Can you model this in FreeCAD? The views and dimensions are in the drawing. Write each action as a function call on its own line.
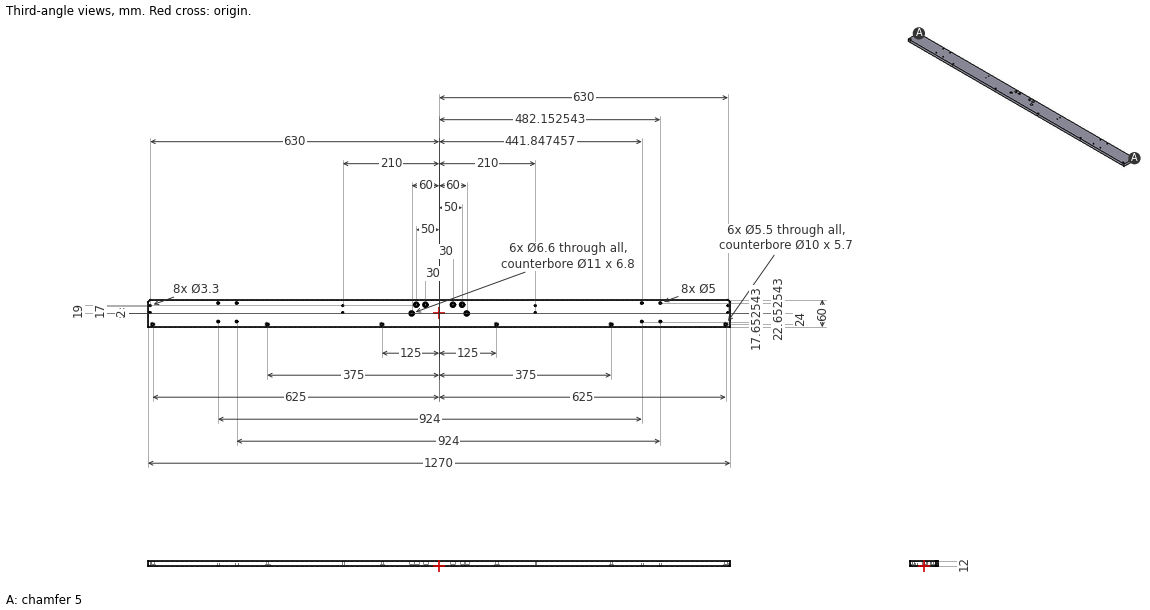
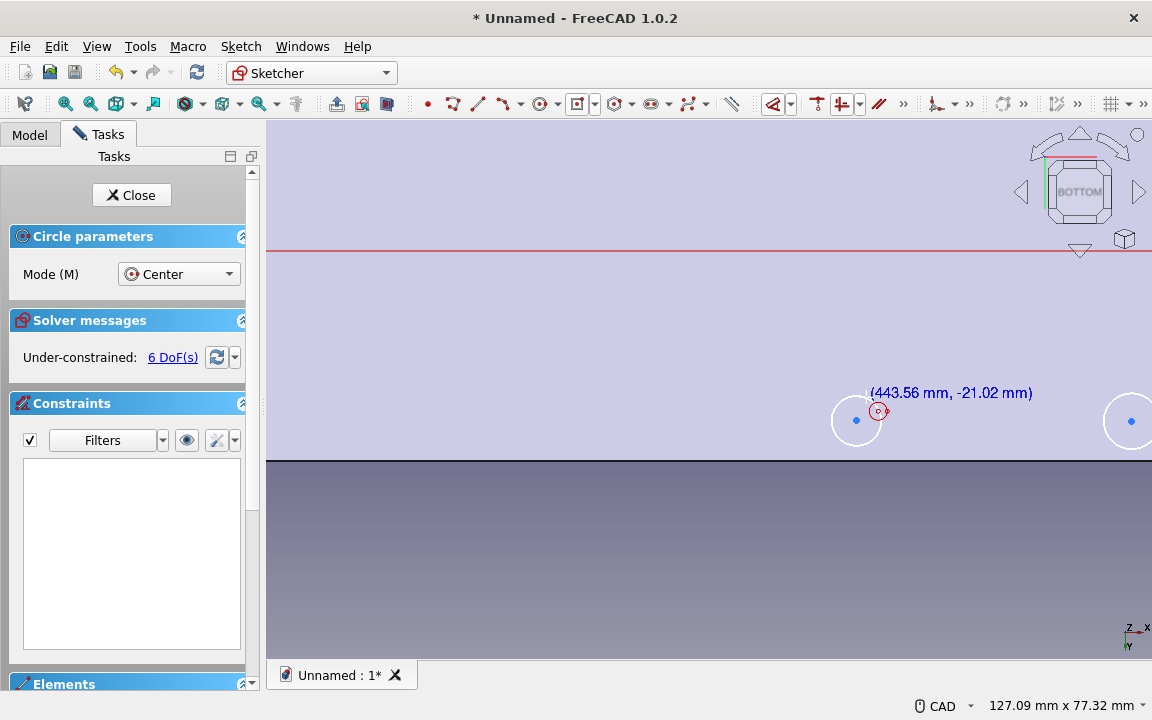
scroll(870, 399, down, 13)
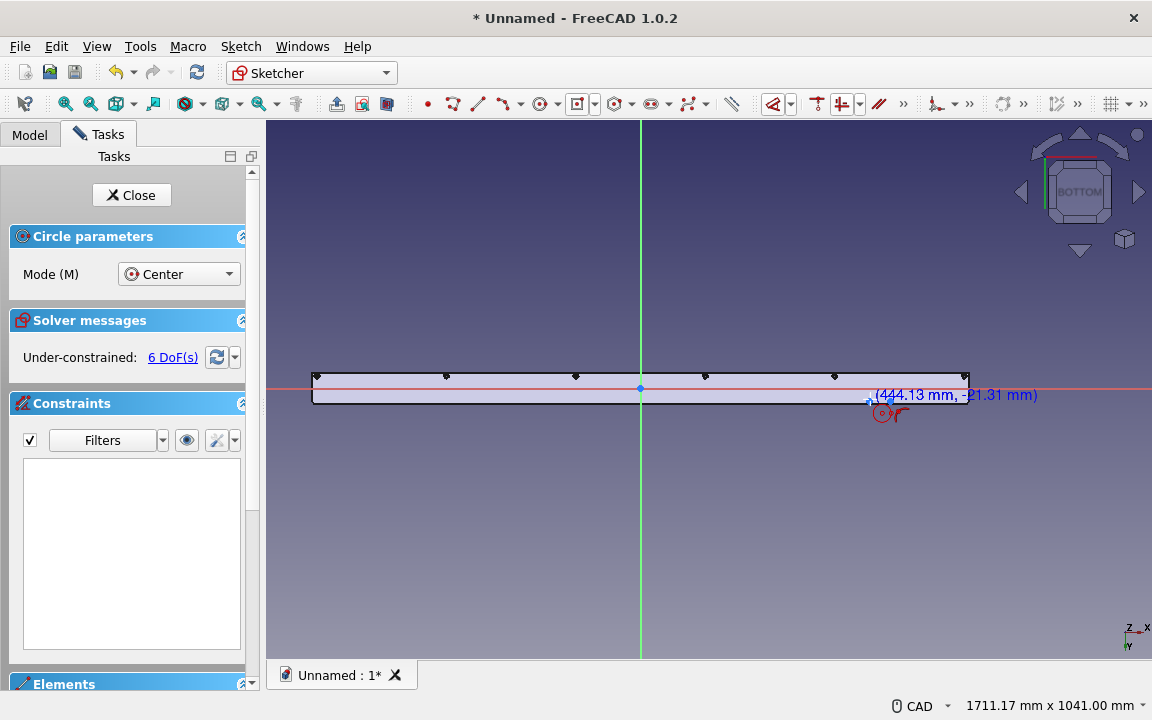
scroll(869, 379, up, 15)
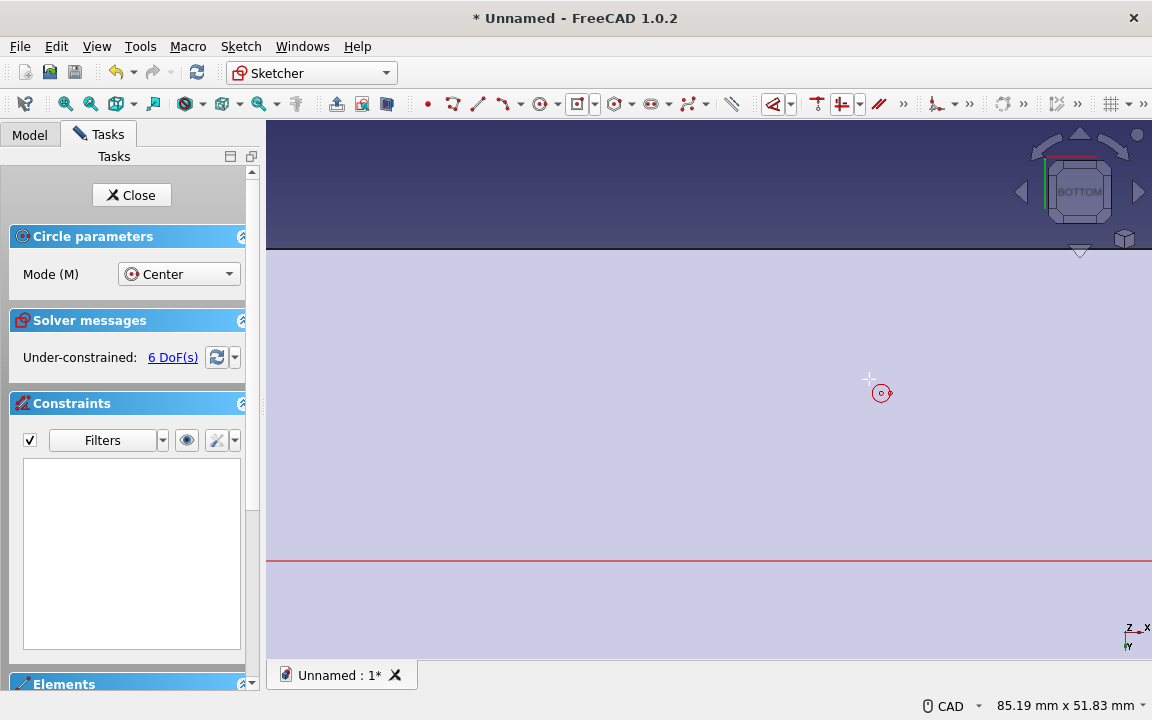
scroll(869, 379, down, 15)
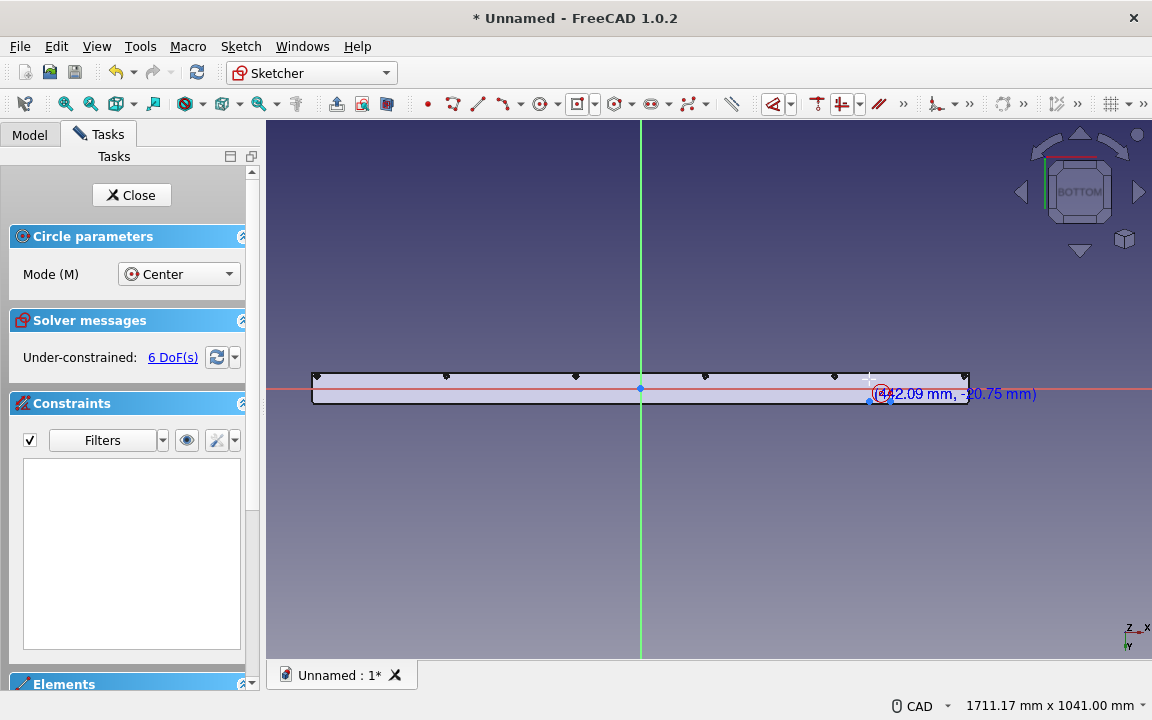
scroll(869, 379, up, 3)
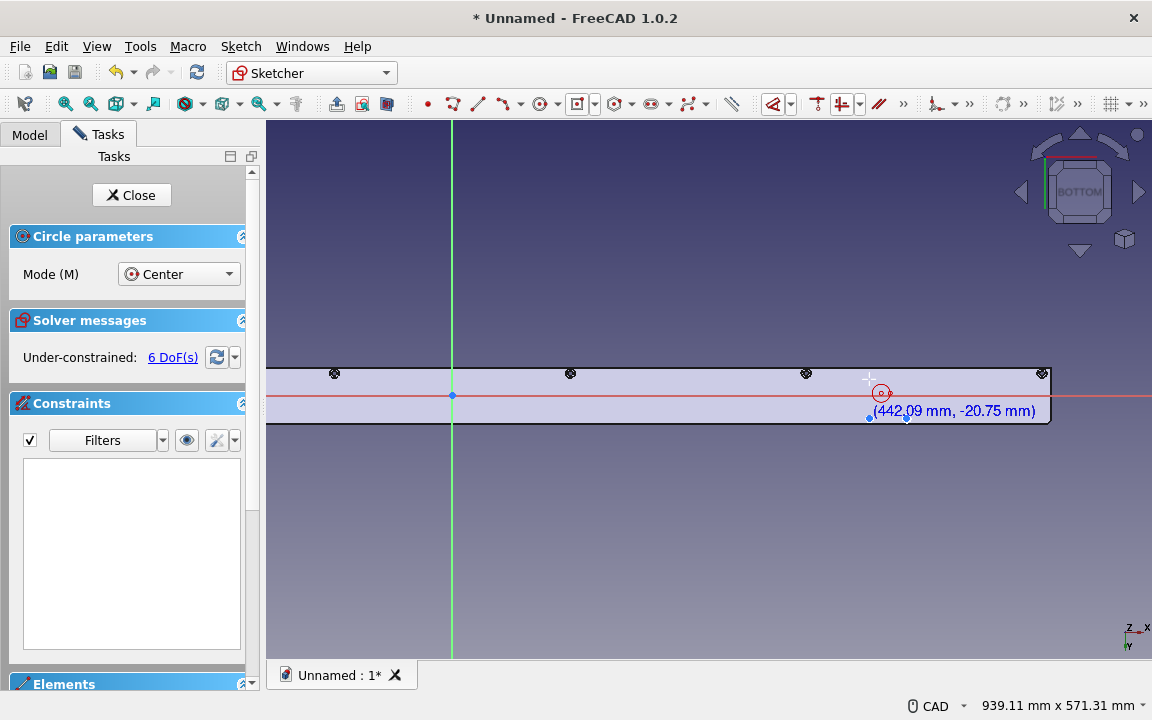
click(869, 379)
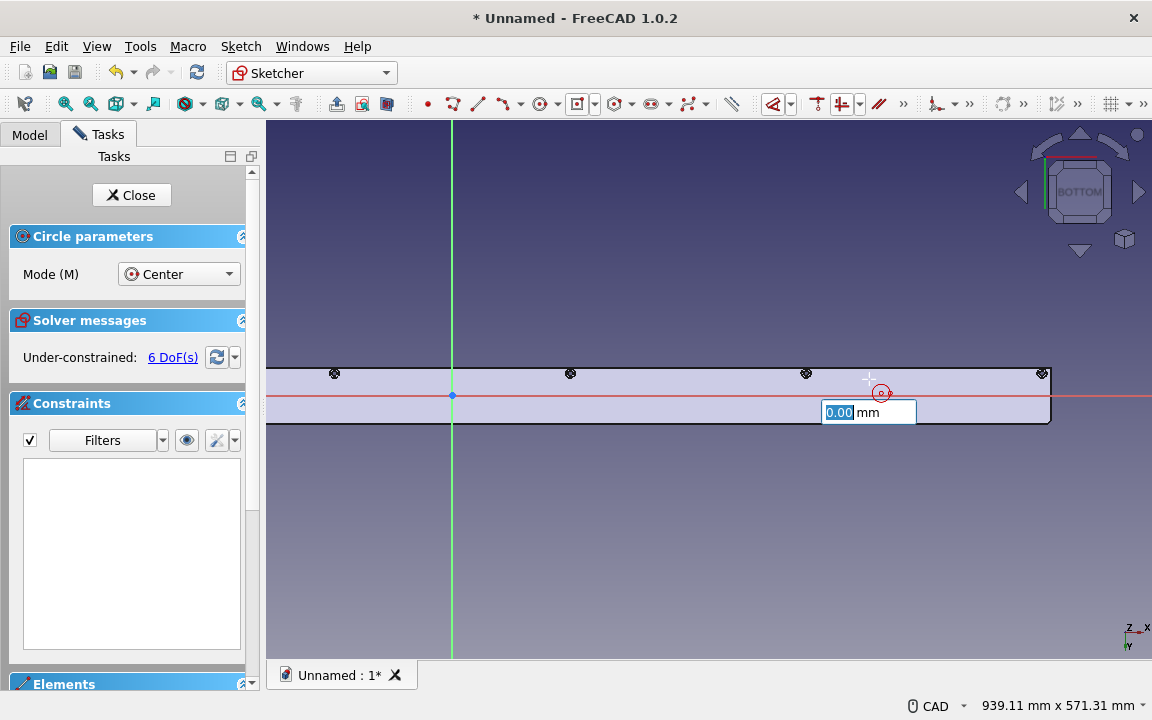
scroll(871, 378, up, 10)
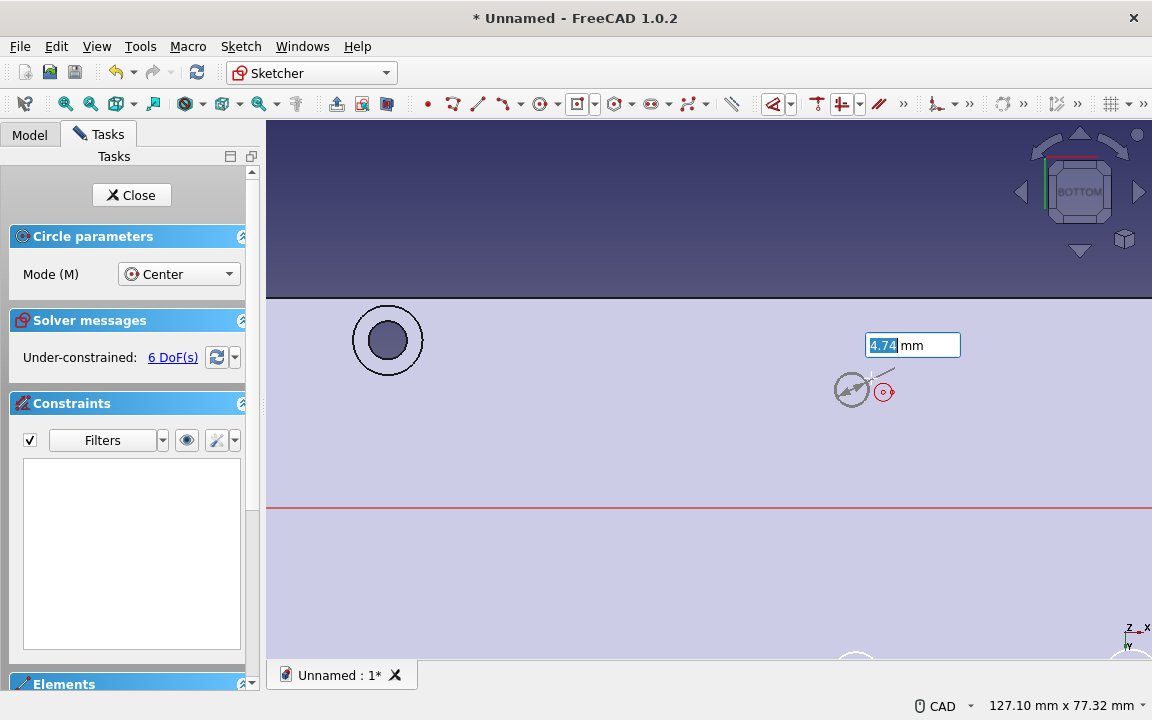
click(866, 372)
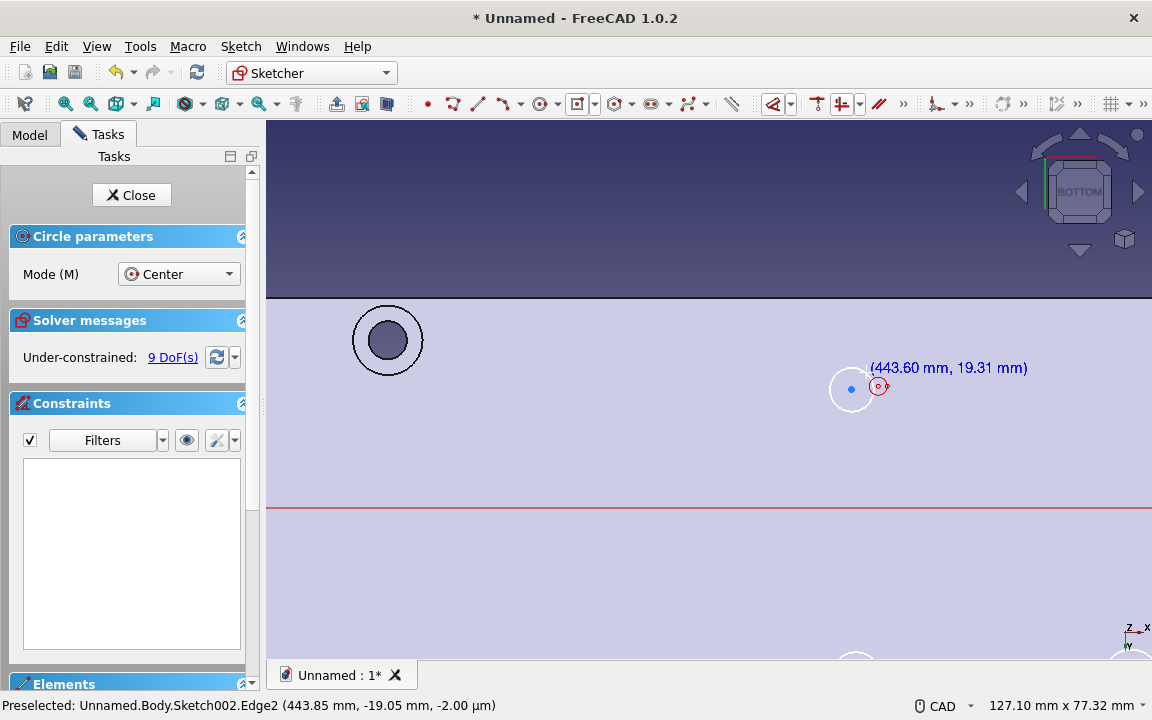
scroll(871, 379, down, 13)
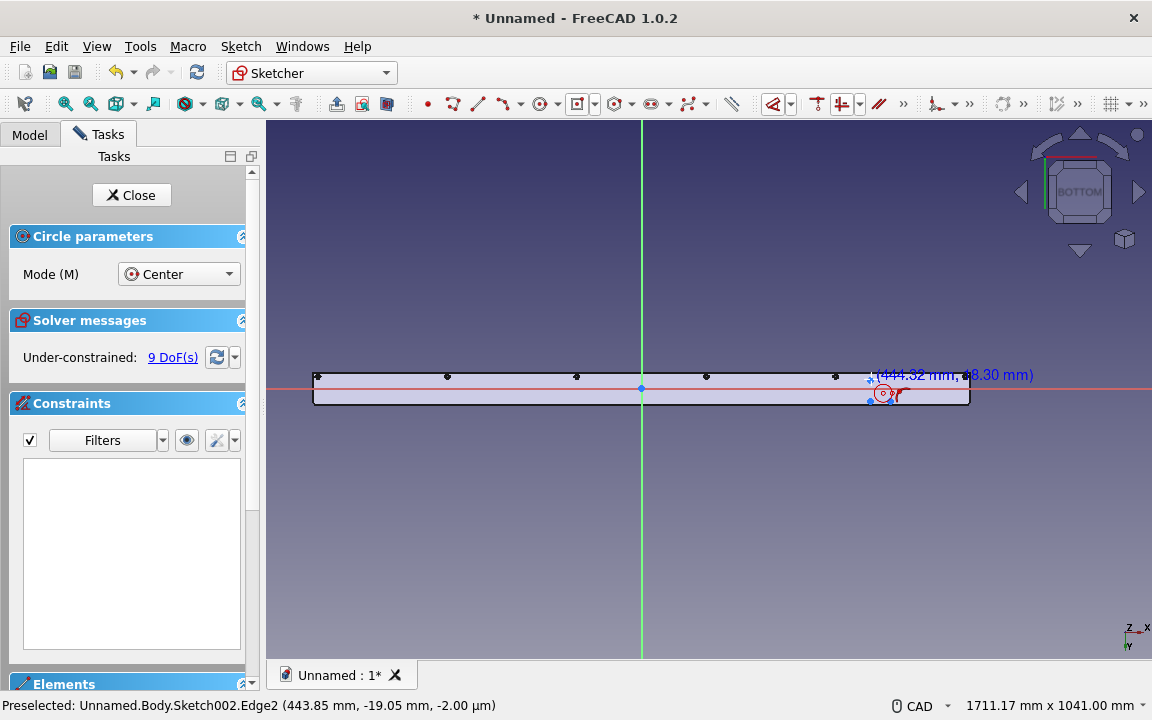
scroll(891, 380, up, 15)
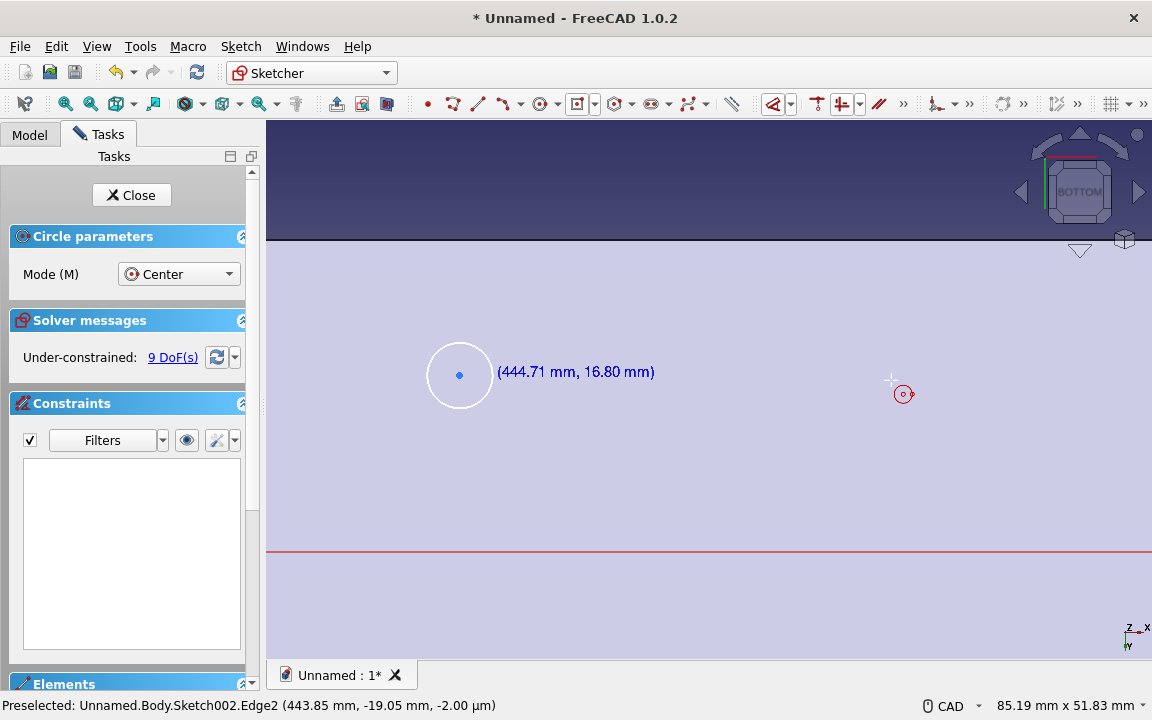
scroll(891, 380, down, 15)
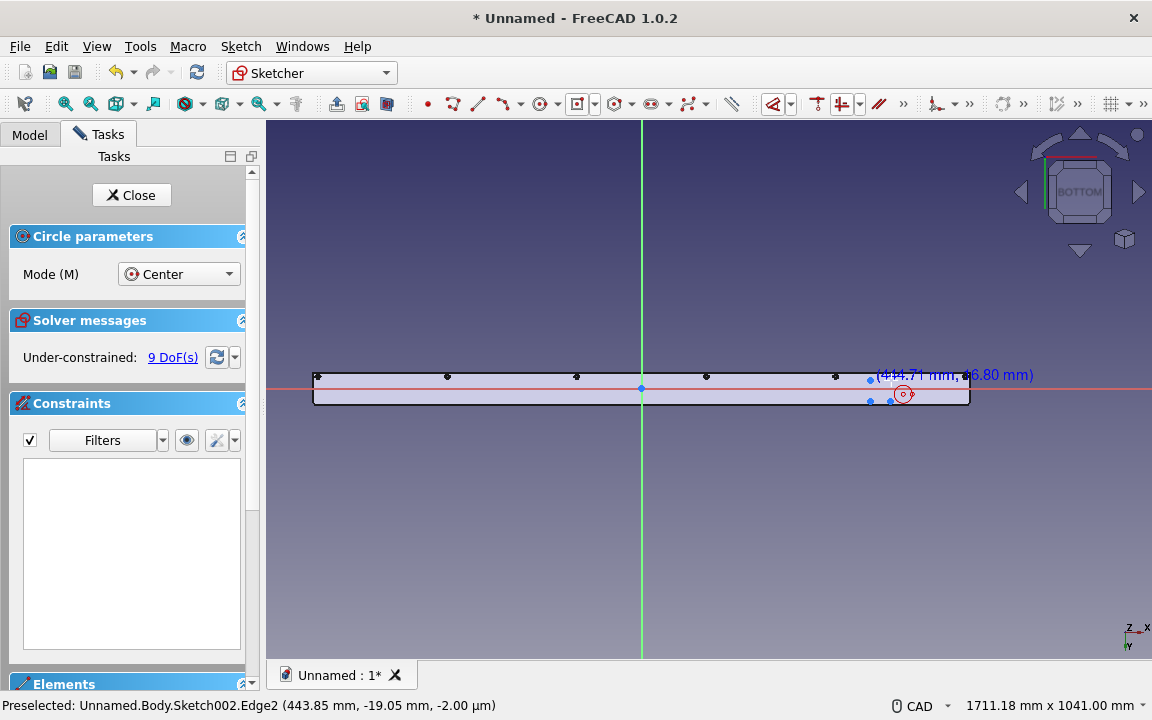
scroll(891, 380, up, 3)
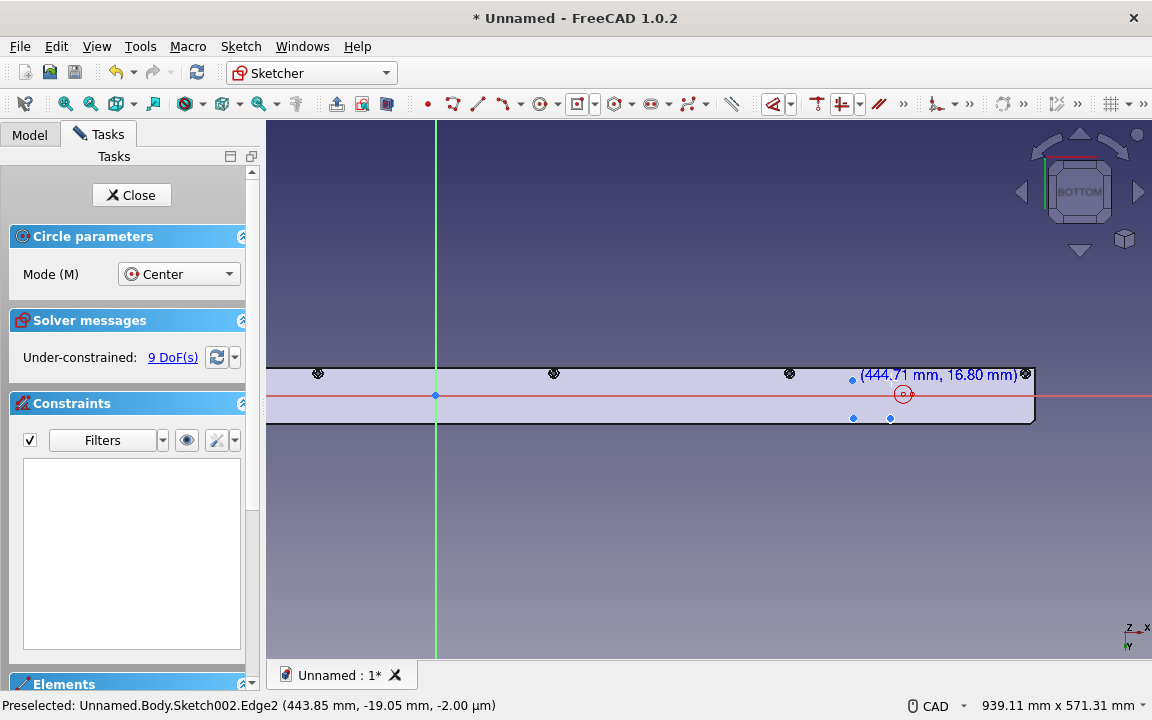
click(891, 379)